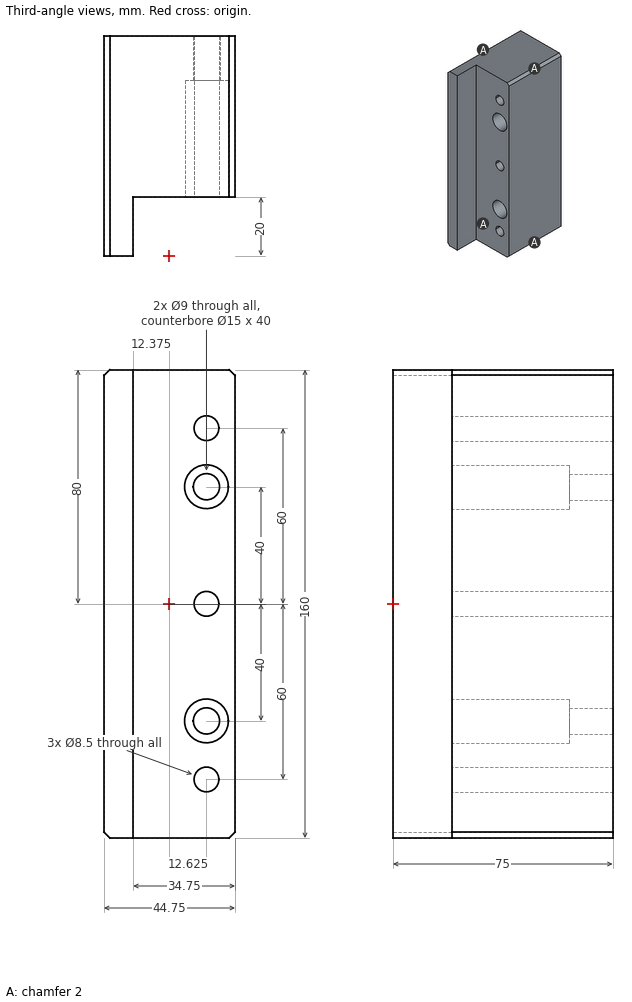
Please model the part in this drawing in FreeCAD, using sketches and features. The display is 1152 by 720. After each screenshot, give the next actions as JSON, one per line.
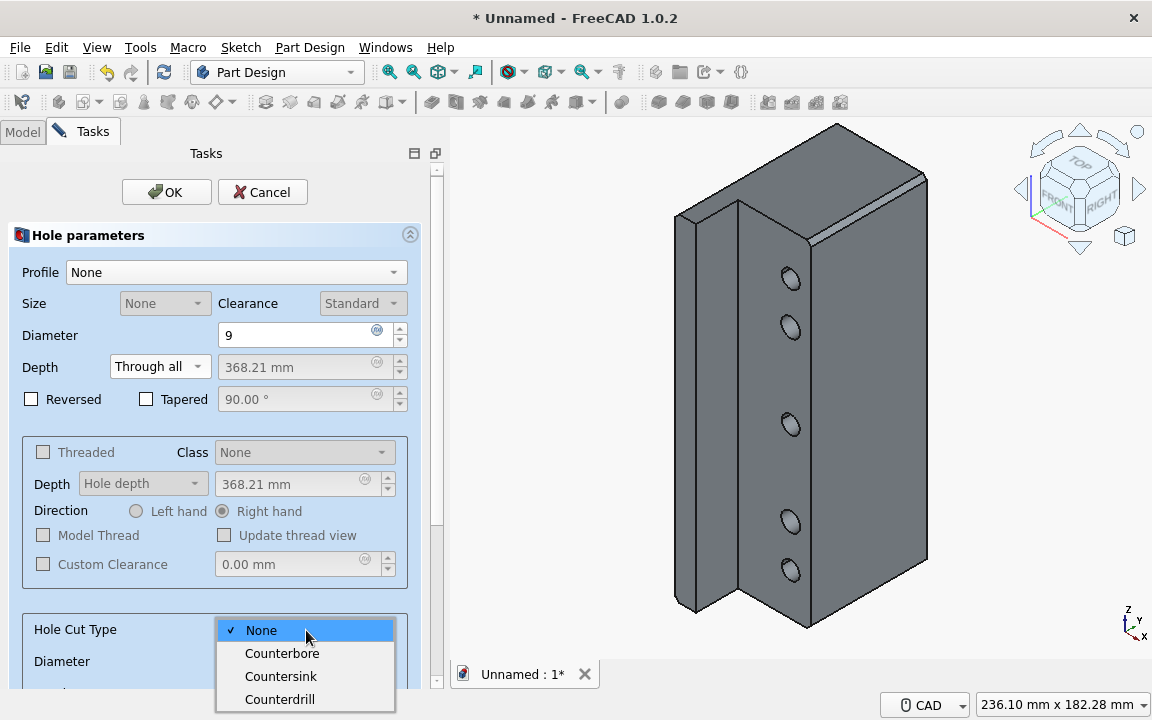
{"action": "left_click", "coordinate": [304, 654]}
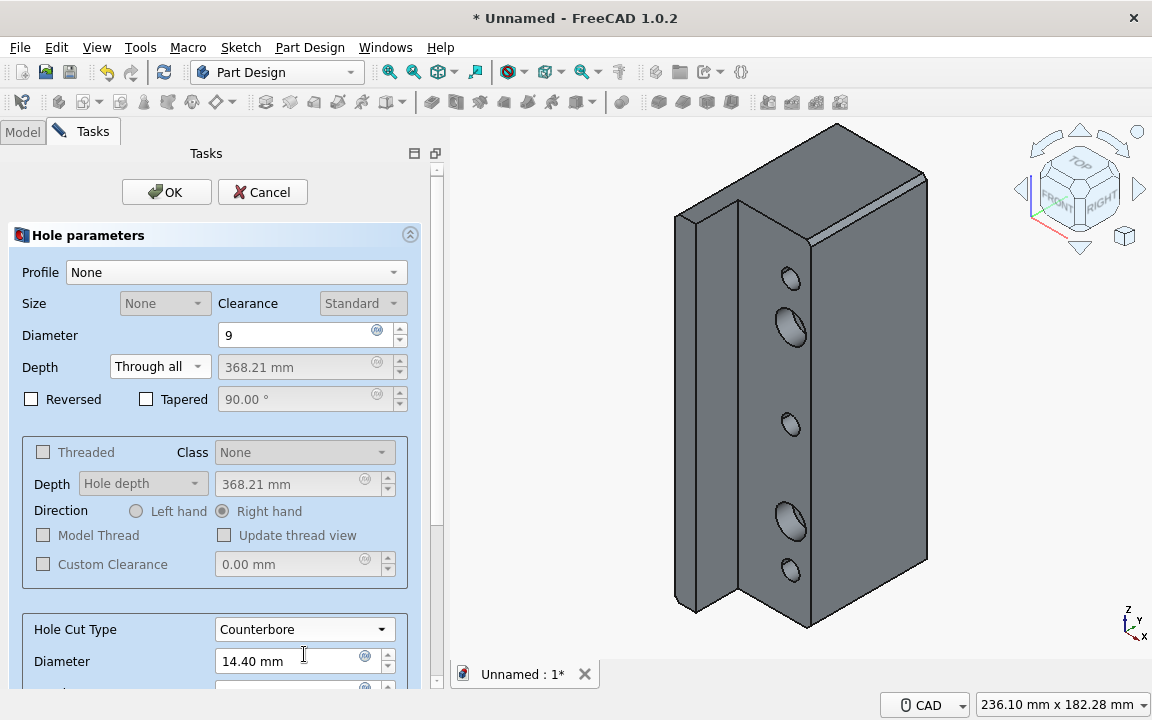
{"action": "triple_click", "coordinate": [298, 661]}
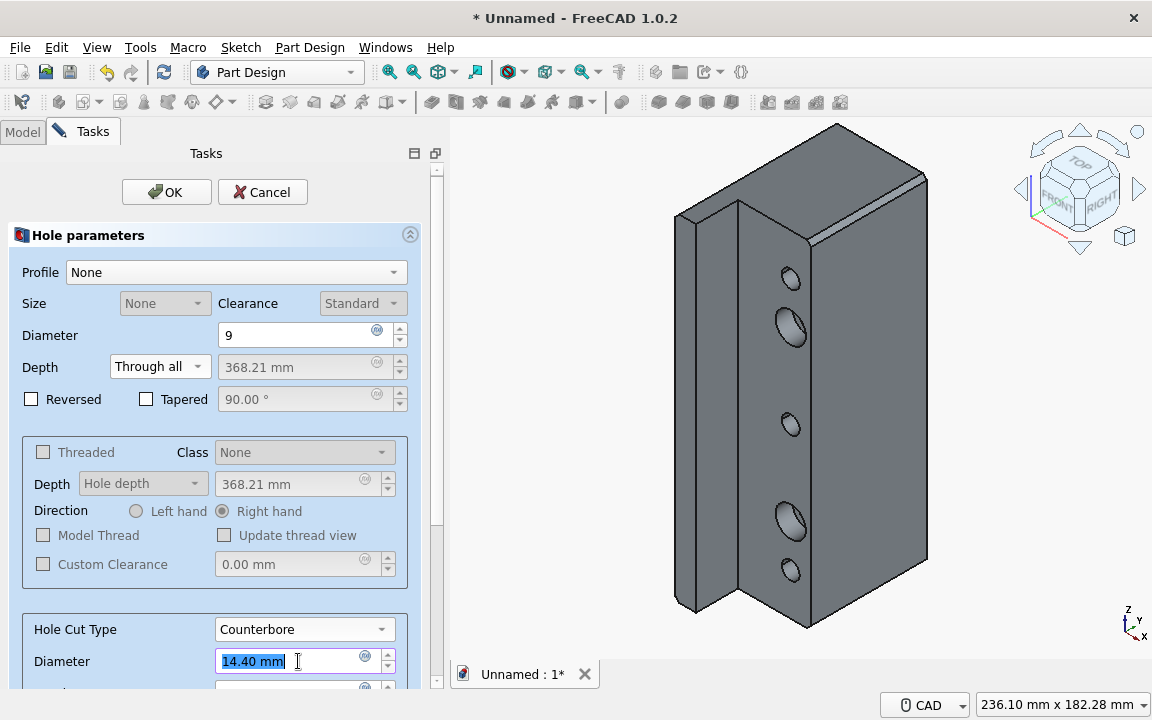
{"action": "type", "text": "15"}
{"action": "key", "text": "Tab"}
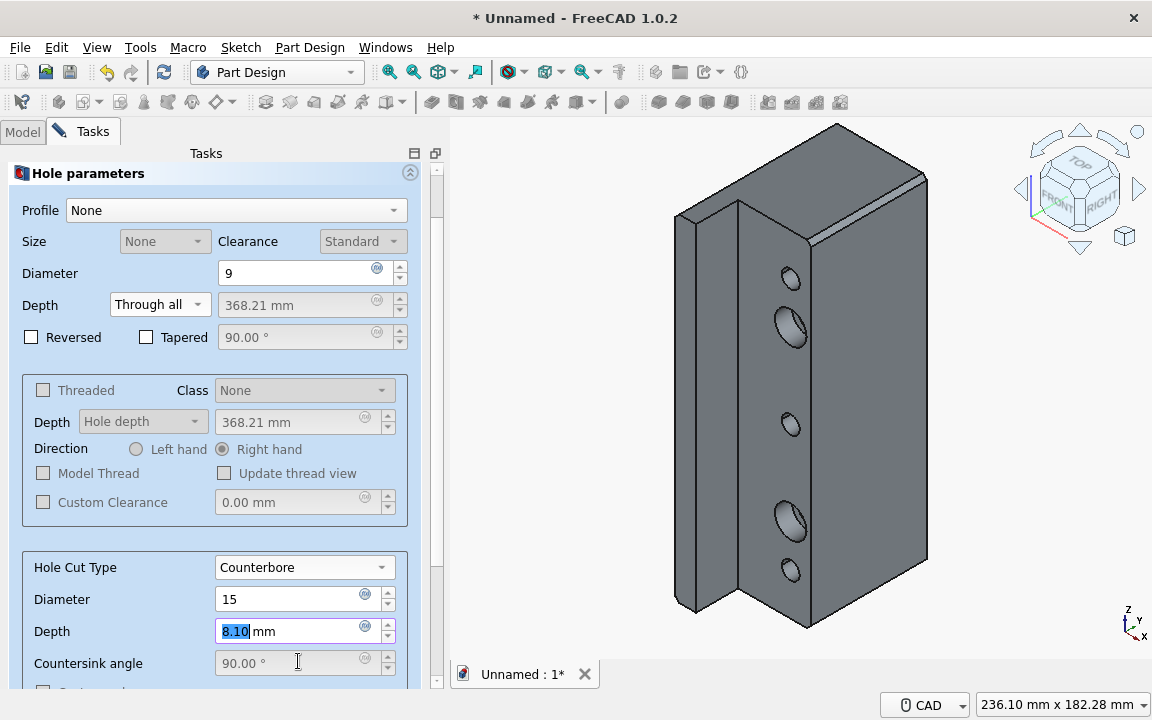
{"action": "type", "text": "40"}
{"action": "key", "text": "Tab"}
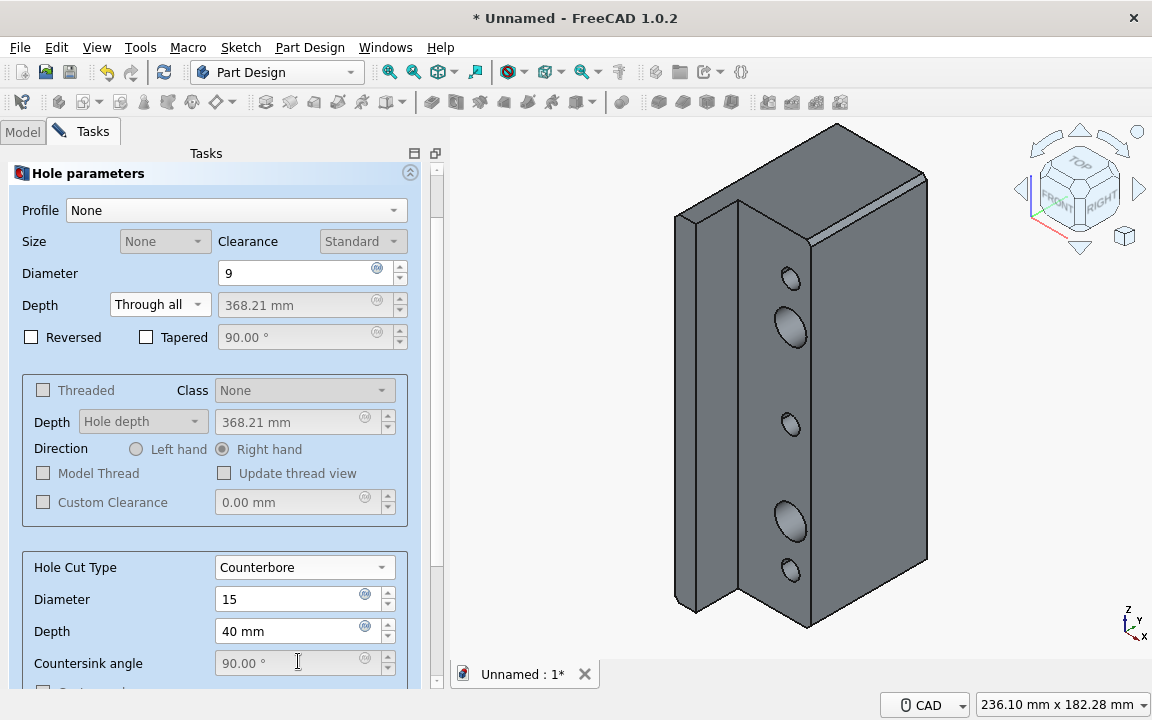
{"action": "scroll", "coordinate": [437, 426], "scroll_direction": "up", "scroll_amount": 2}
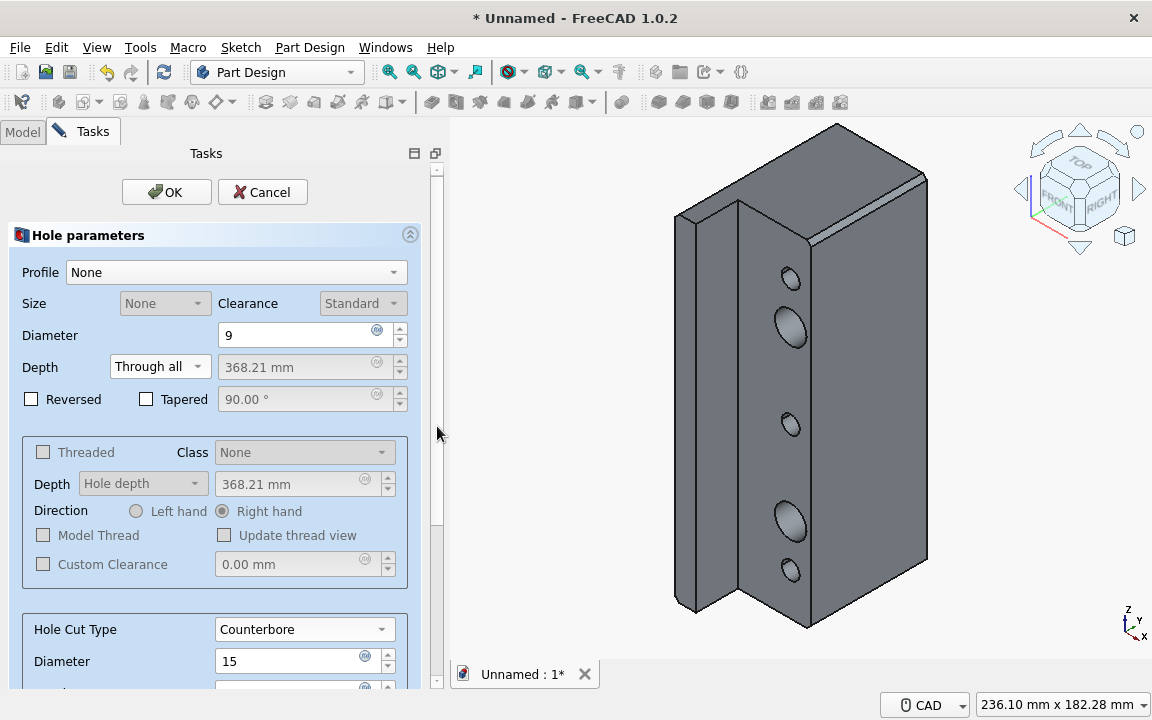
{"action": "left_click", "coordinate": [167, 192]}